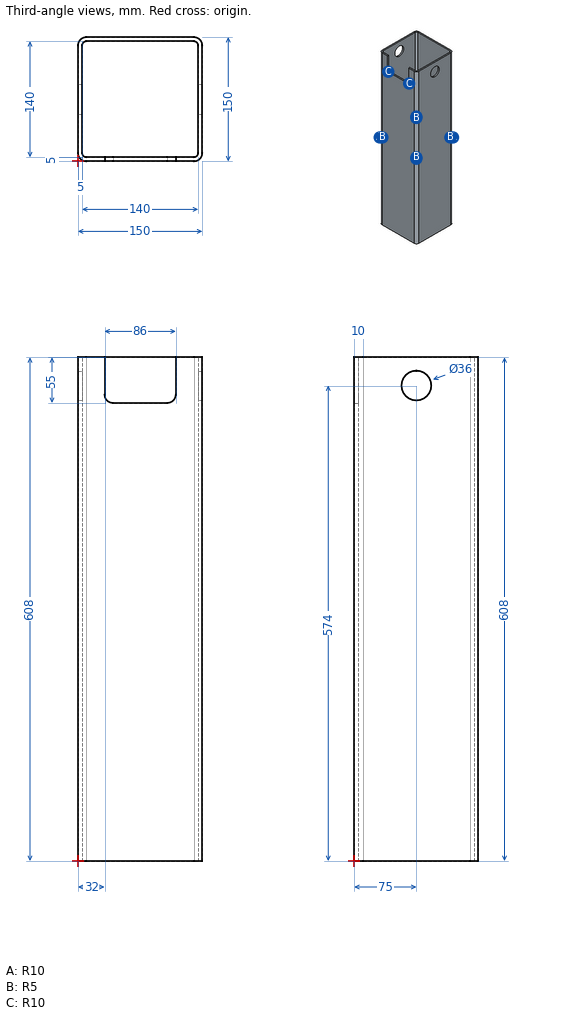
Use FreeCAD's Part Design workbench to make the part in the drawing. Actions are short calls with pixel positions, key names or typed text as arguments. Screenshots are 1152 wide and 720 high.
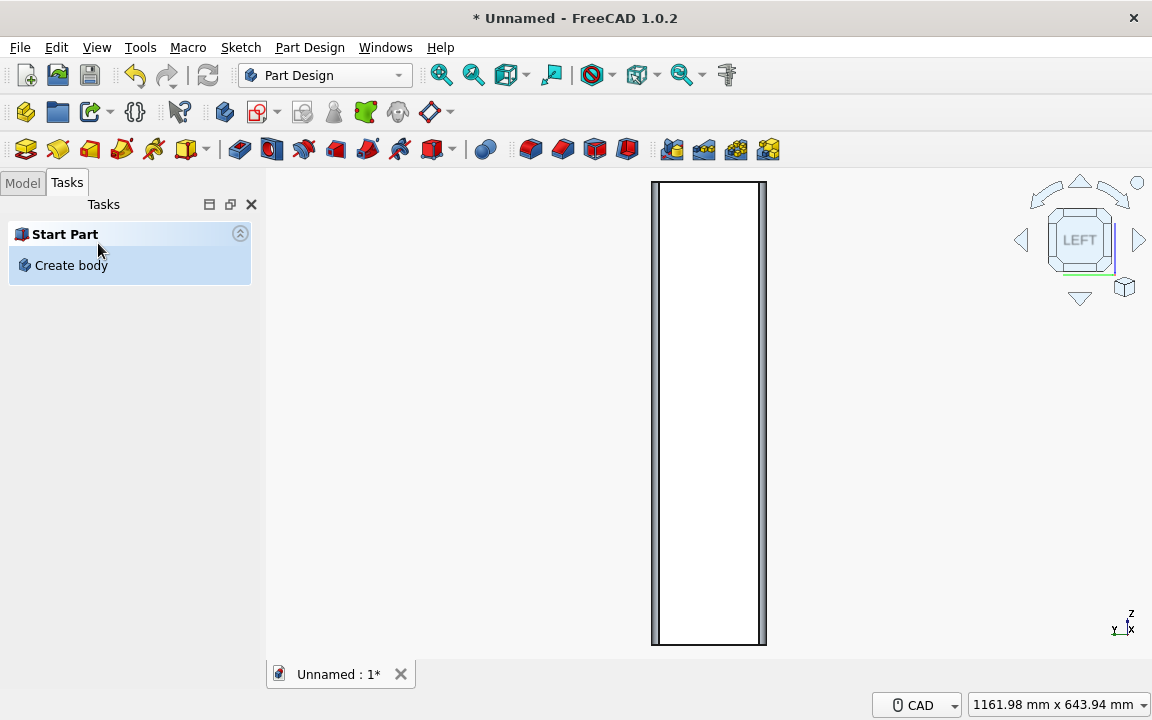
click(709, 280)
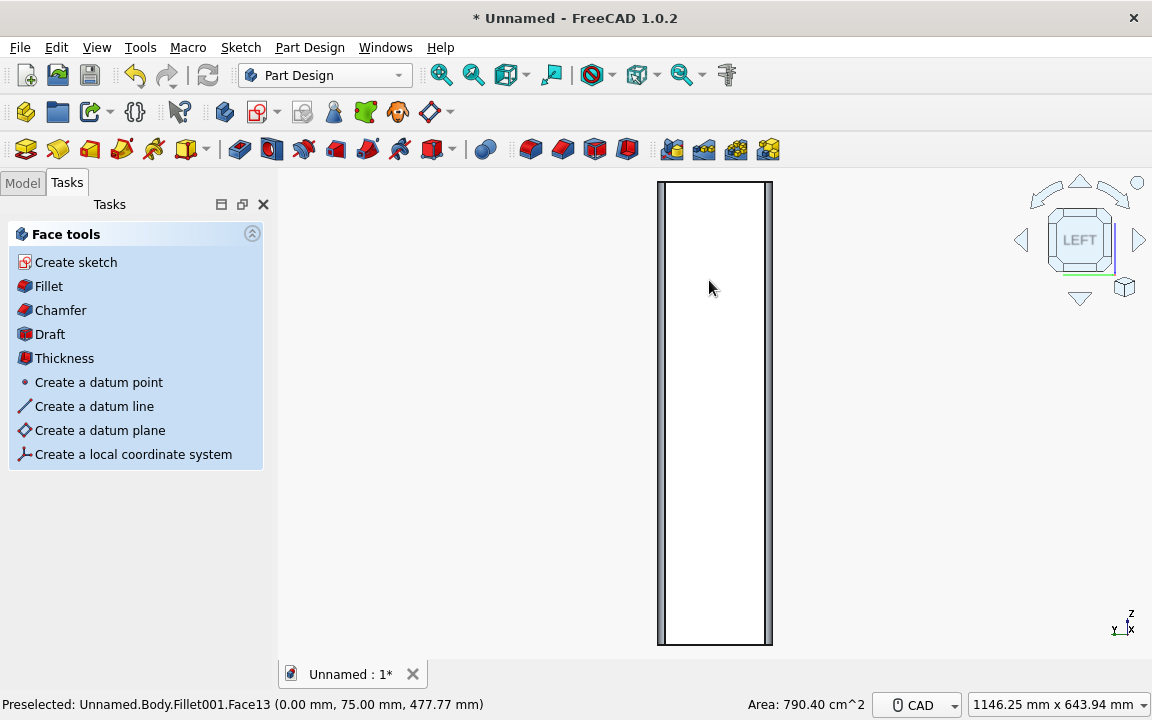
click(258, 112)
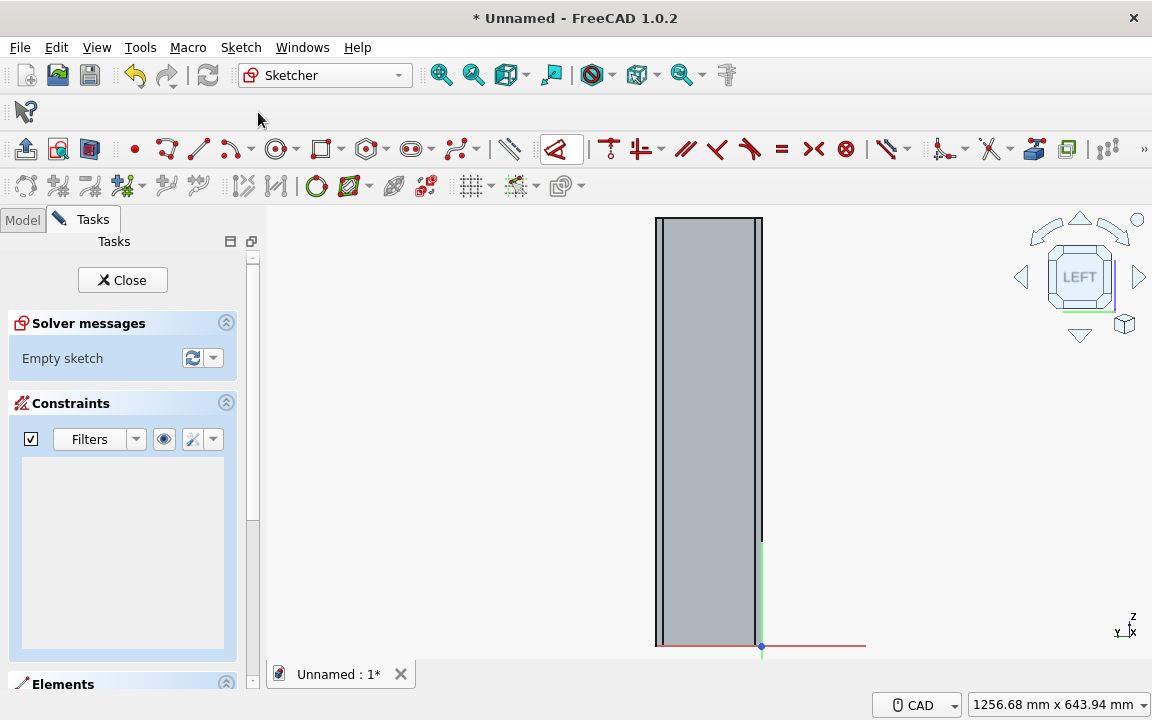
scroll(640, 432, down, 5)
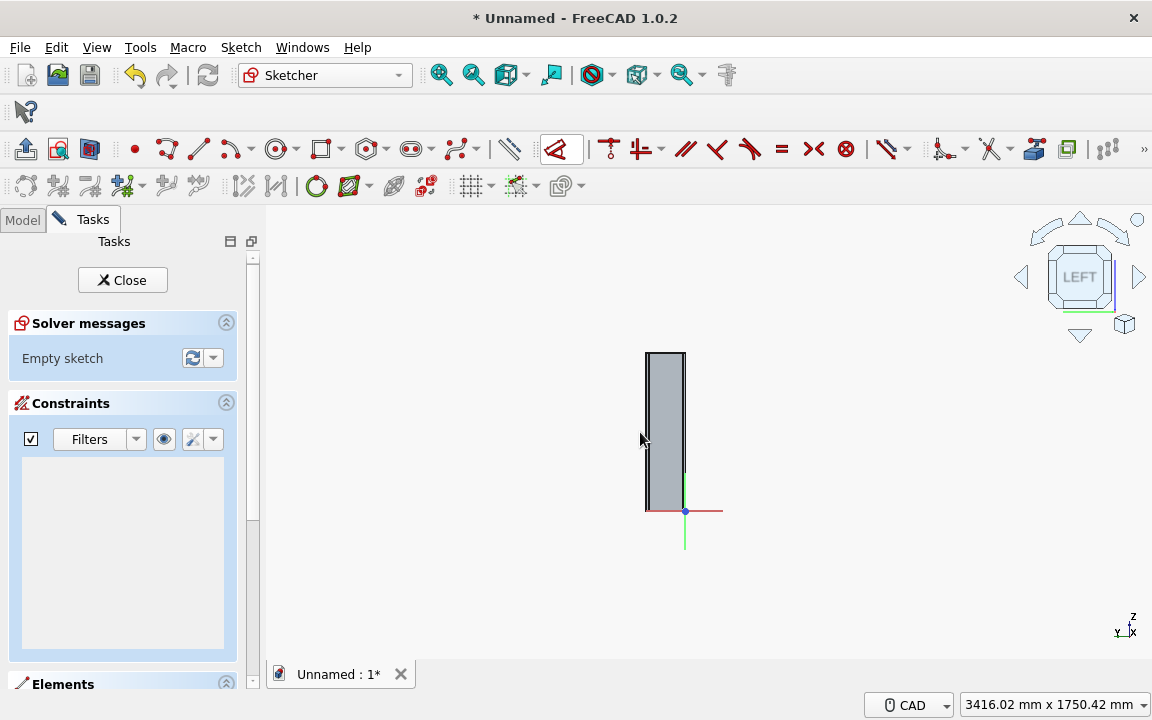
scroll(667, 359, up, 15)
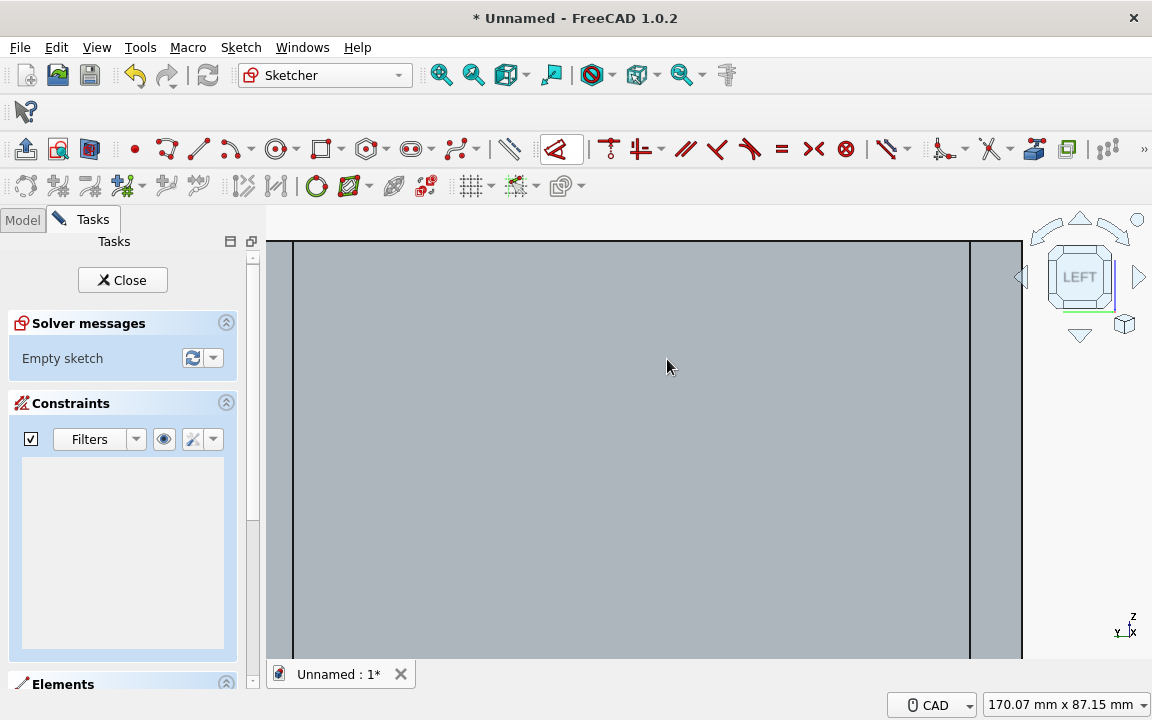
scroll(612, 391, up, 2)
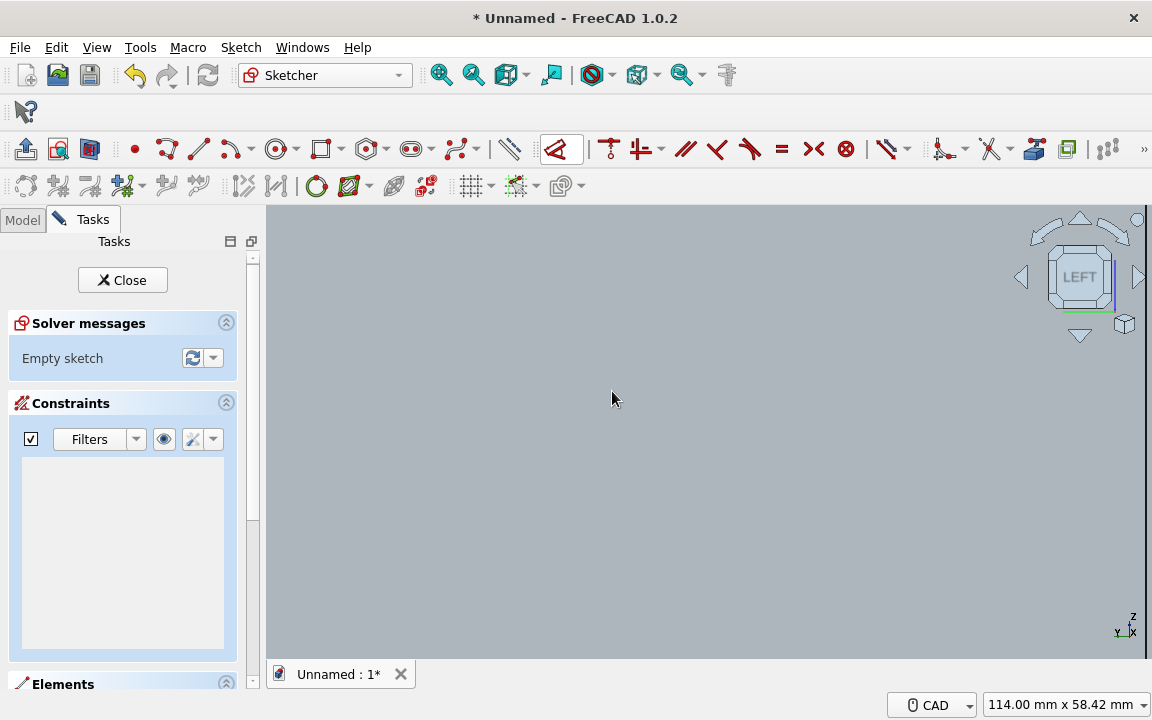
click(276, 150)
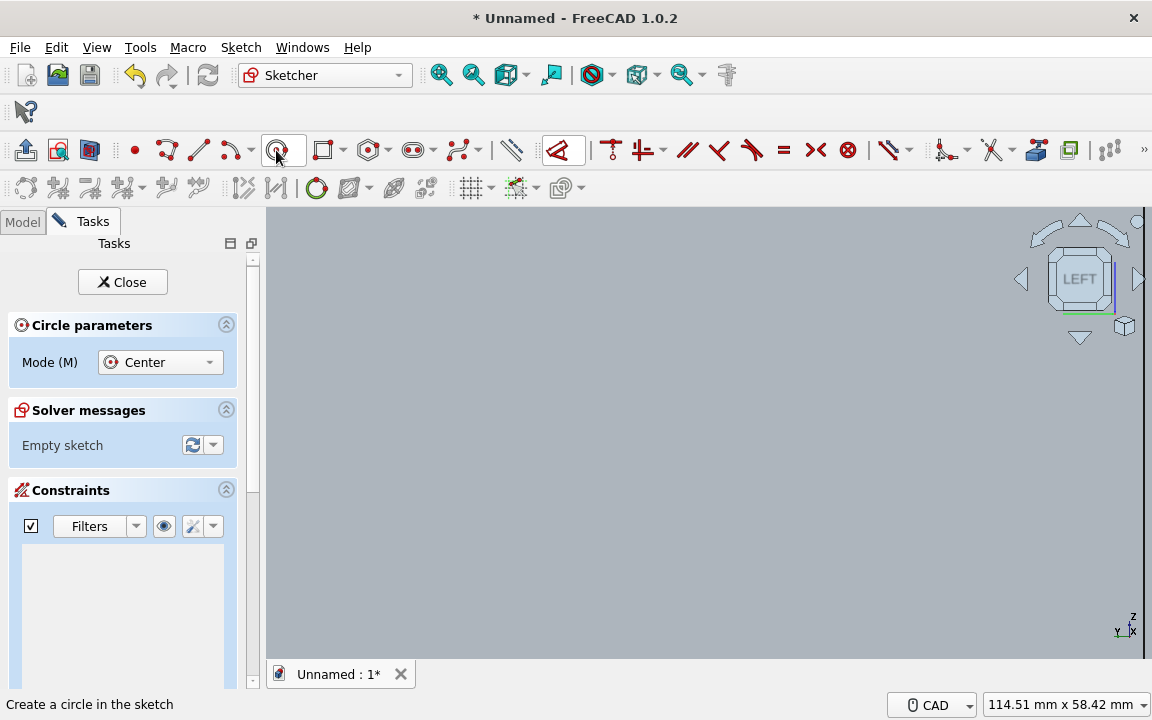
click(641, 433)
click(739, 334)
key(Escape)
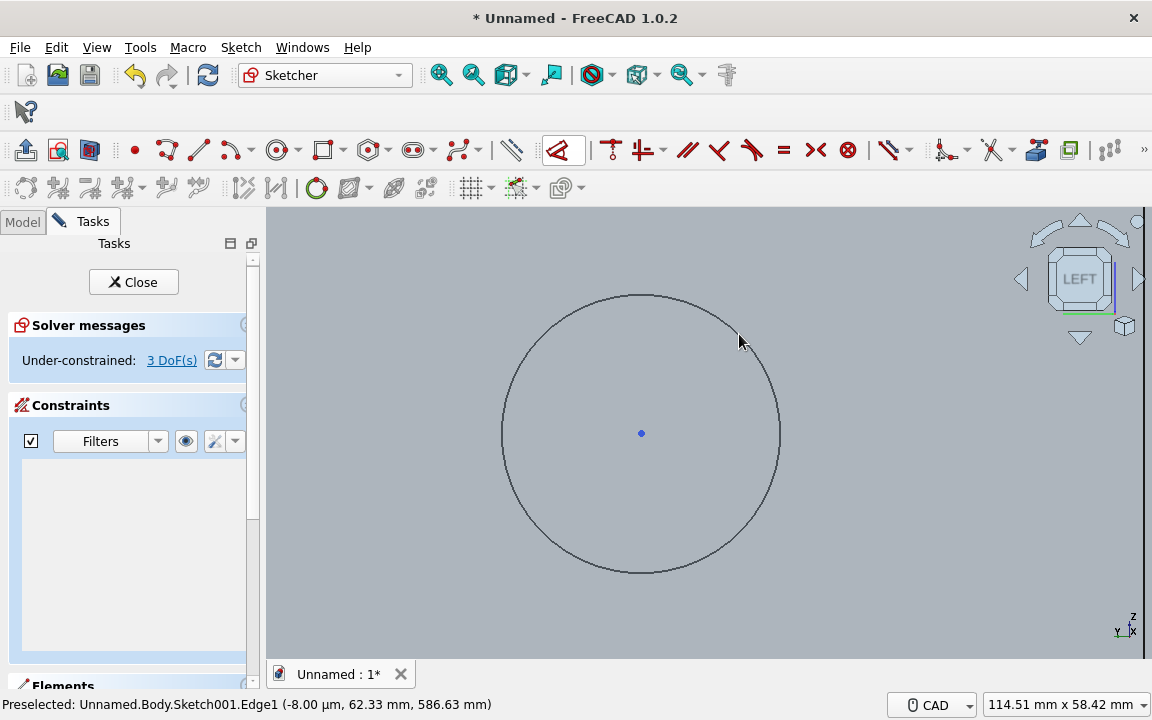
click(739, 335)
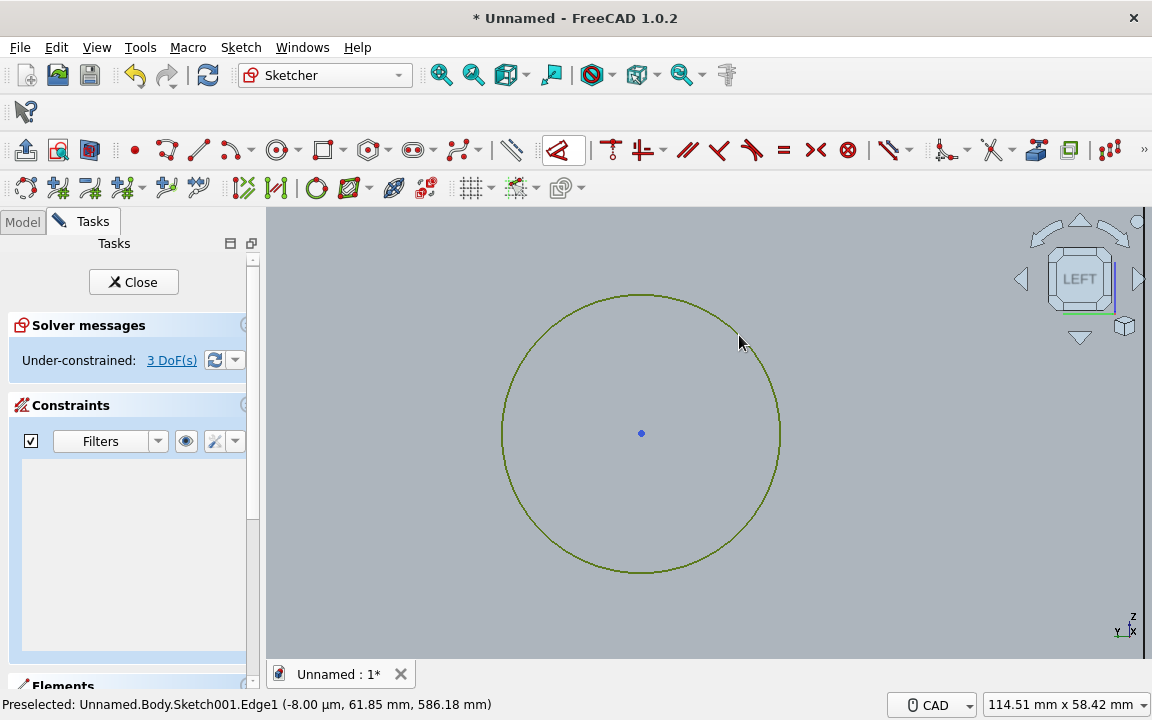
key(k)
key(o)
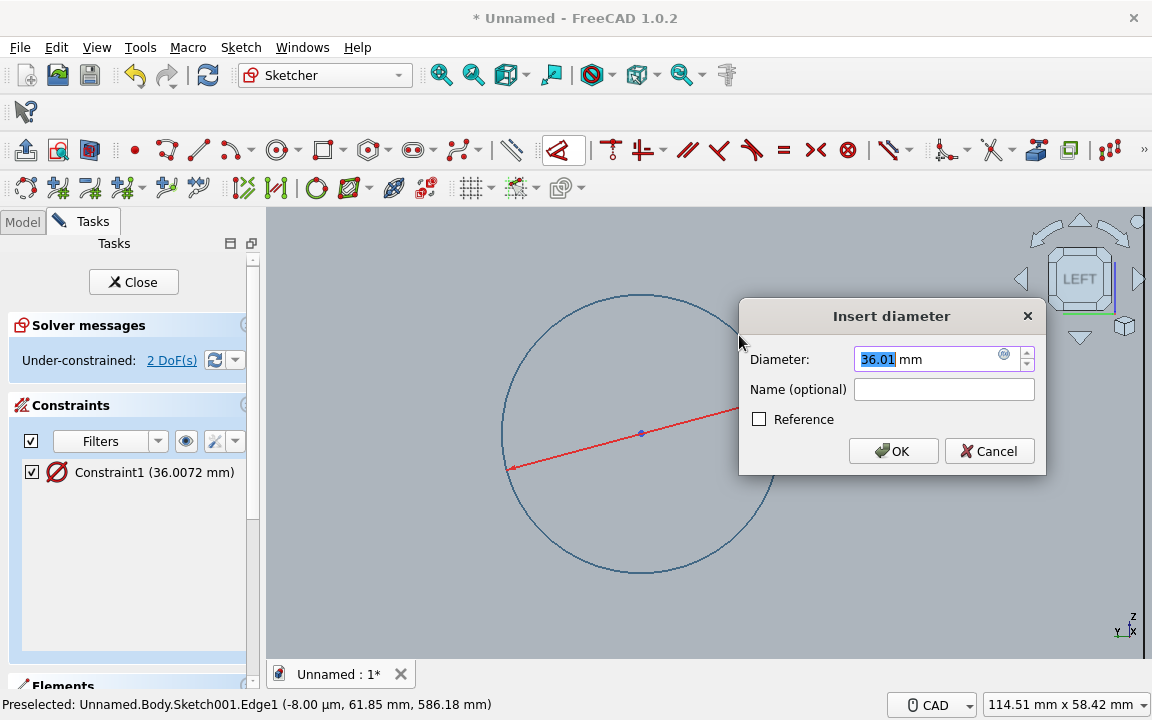
text(36)
key(Return)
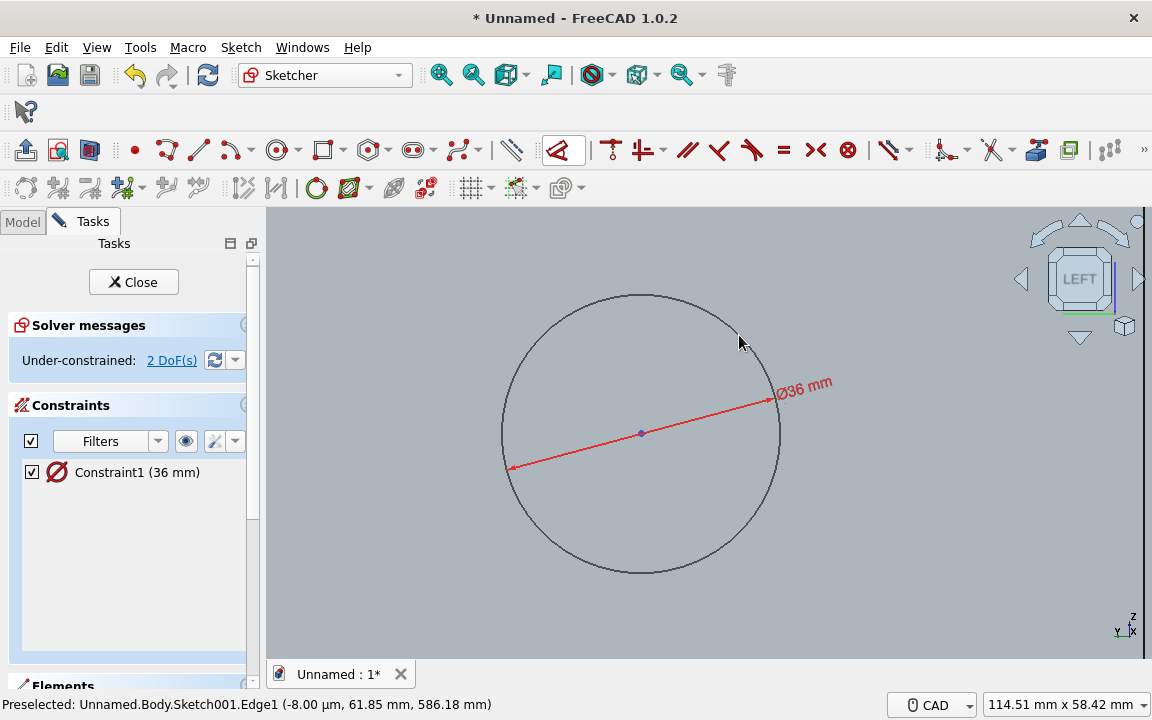
click(641, 434)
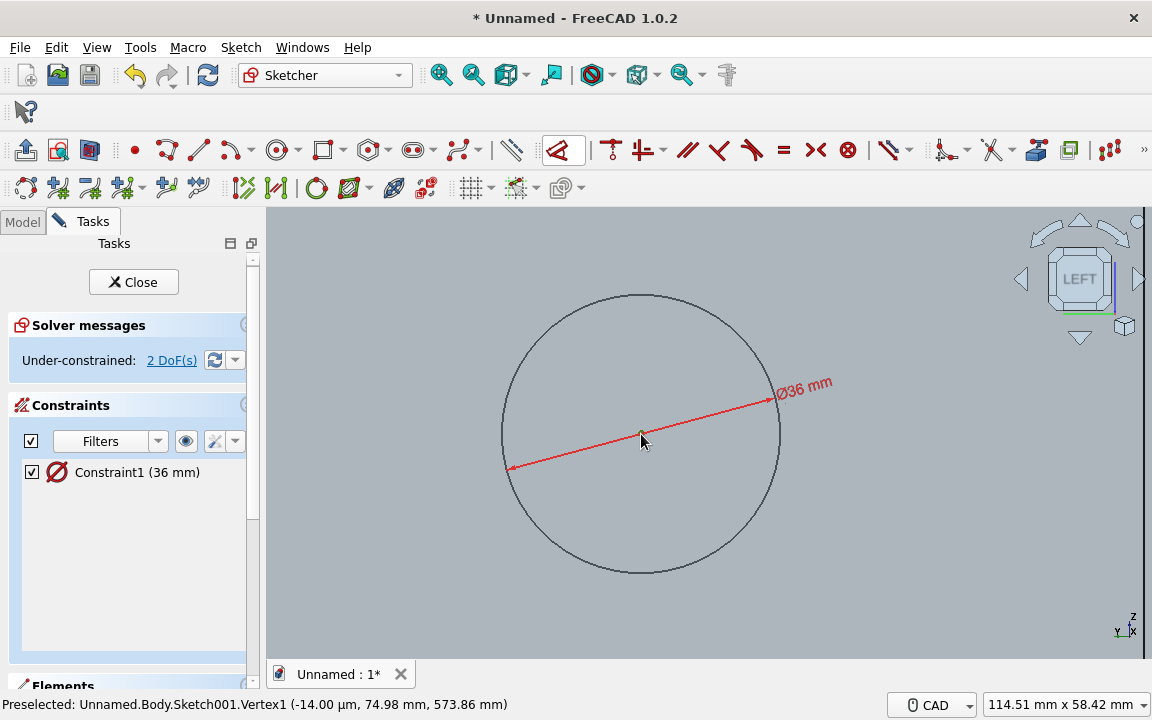
click(580, 150)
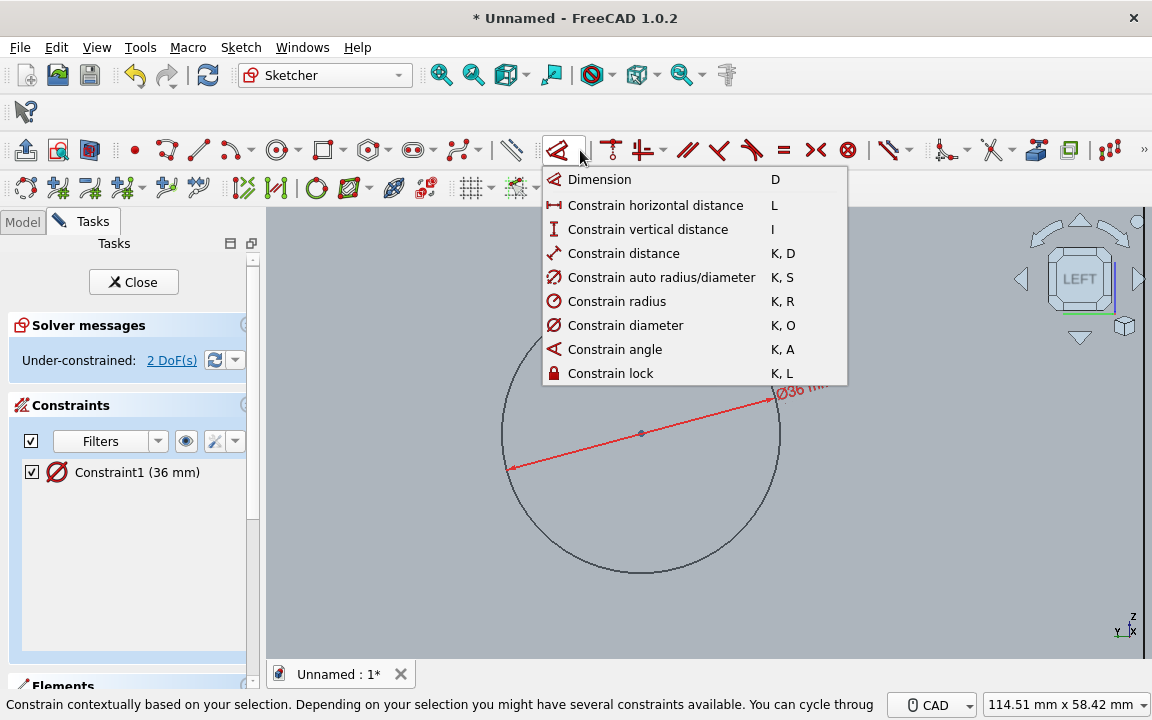
click(695, 205)